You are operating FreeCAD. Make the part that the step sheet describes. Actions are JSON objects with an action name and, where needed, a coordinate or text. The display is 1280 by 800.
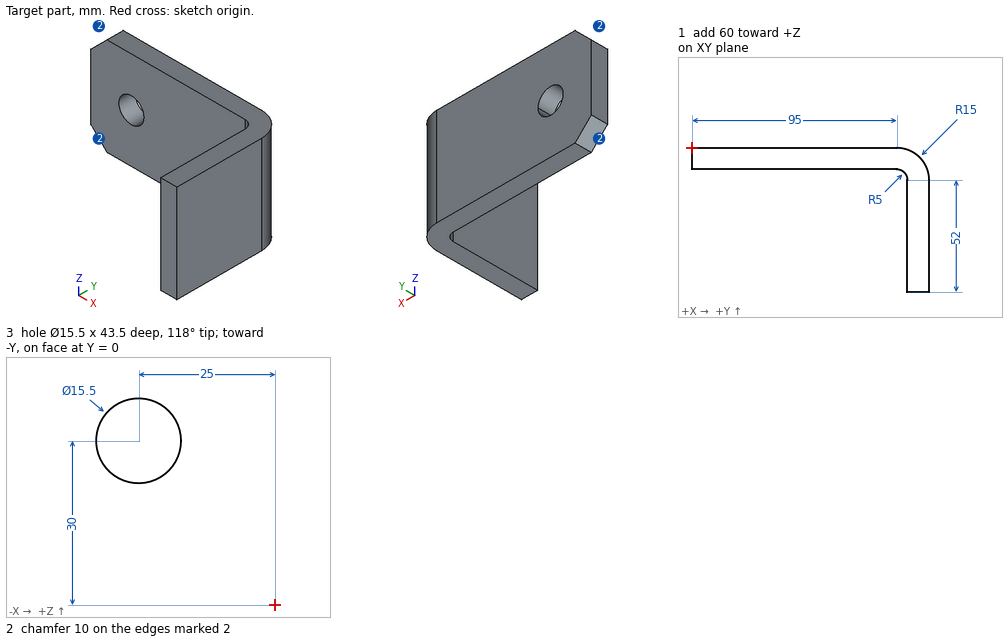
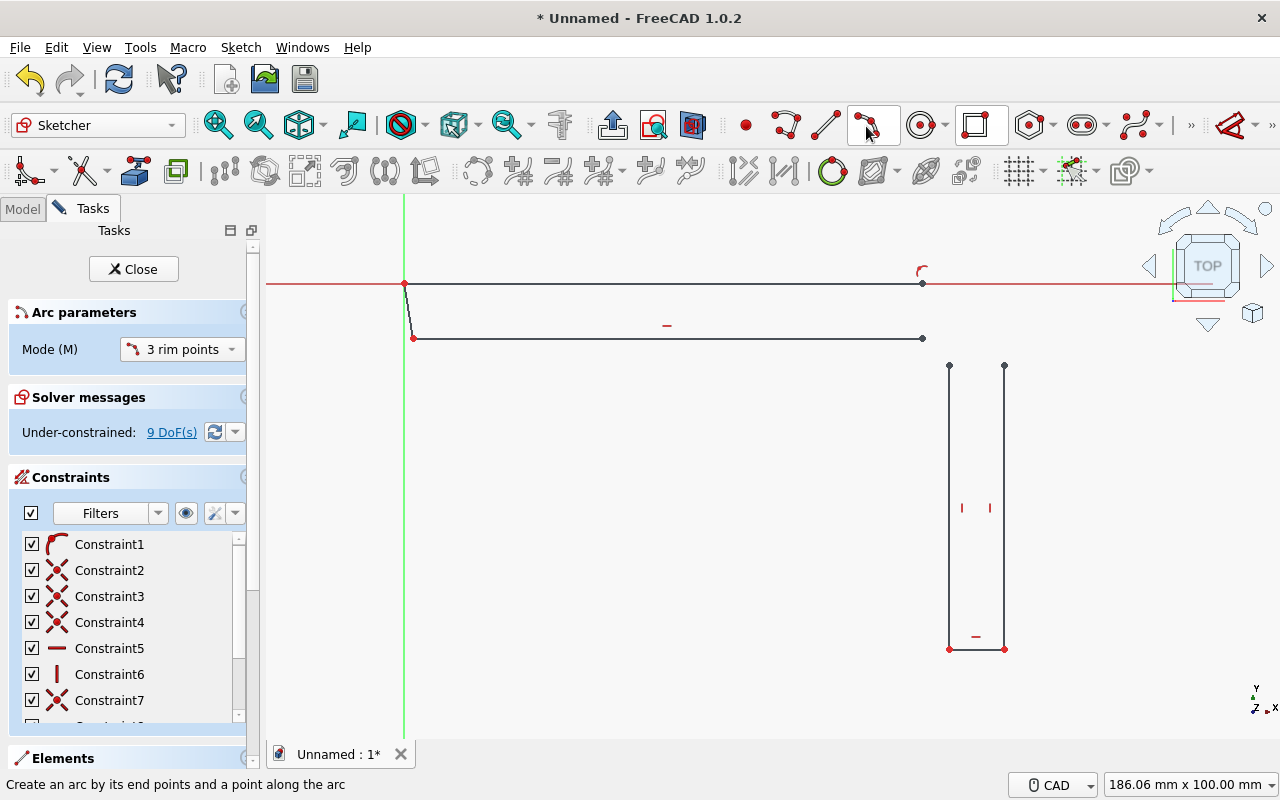
{"action": "left_click", "coordinate": [922, 339]}
{"action": "left_click", "coordinate": [949, 366]}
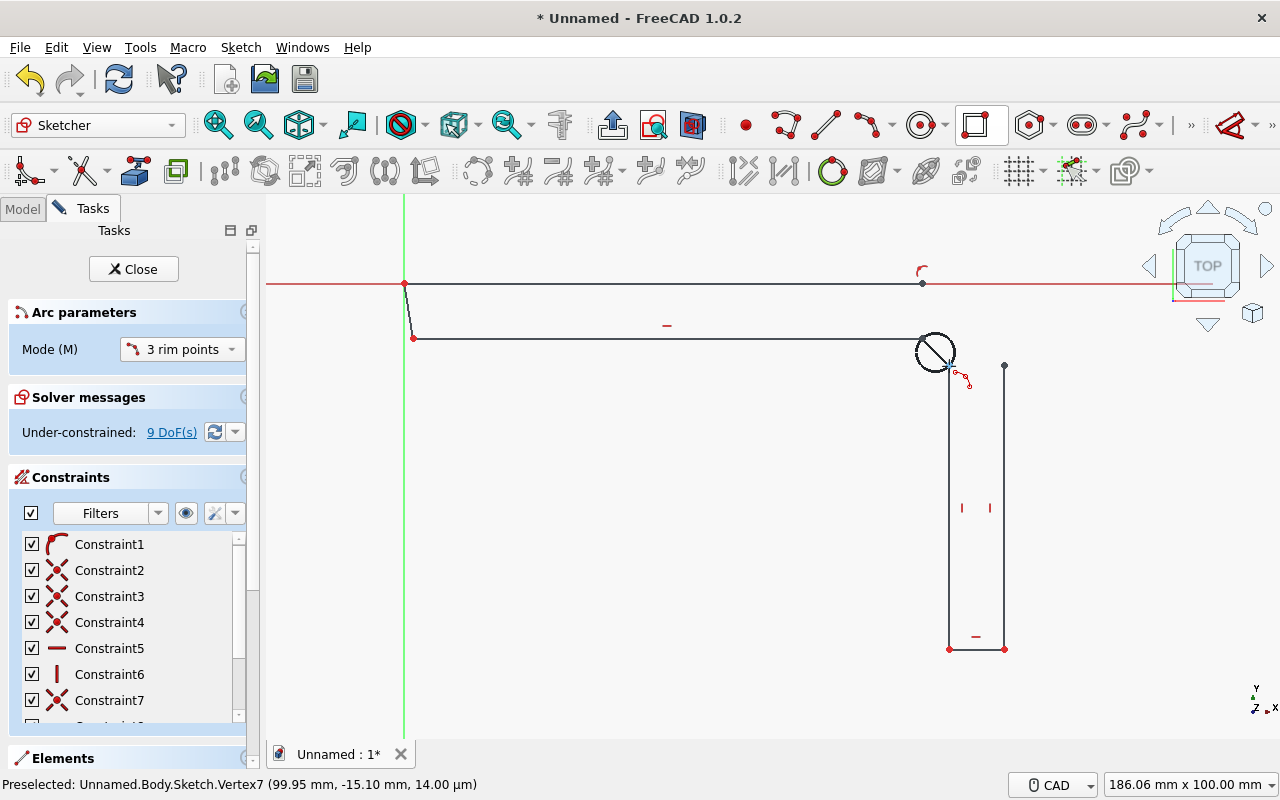
{"action": "scroll", "coordinate": [941, 346], "scroll_direction": "up", "scroll_amount": 4}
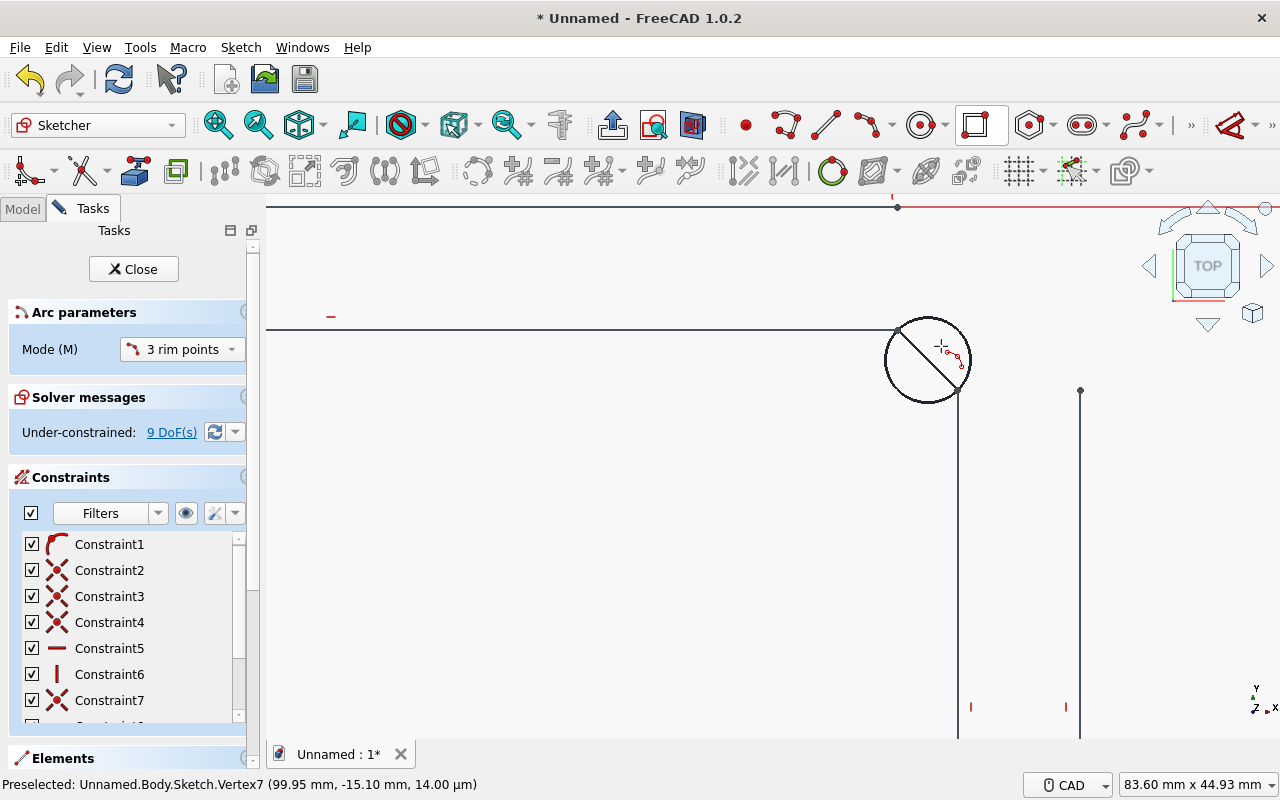
{"action": "left_click", "coordinate": [941, 346]}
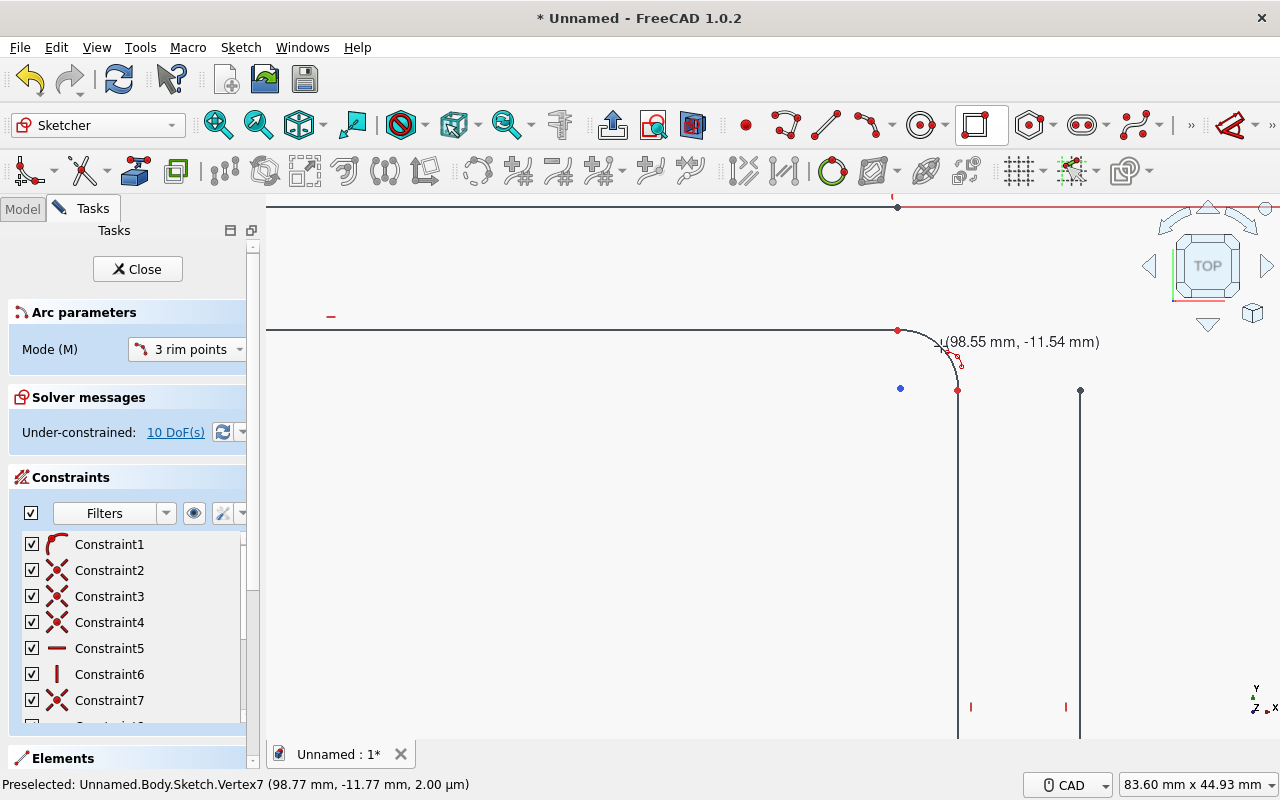
{"action": "left_click", "coordinate": [1080, 390]}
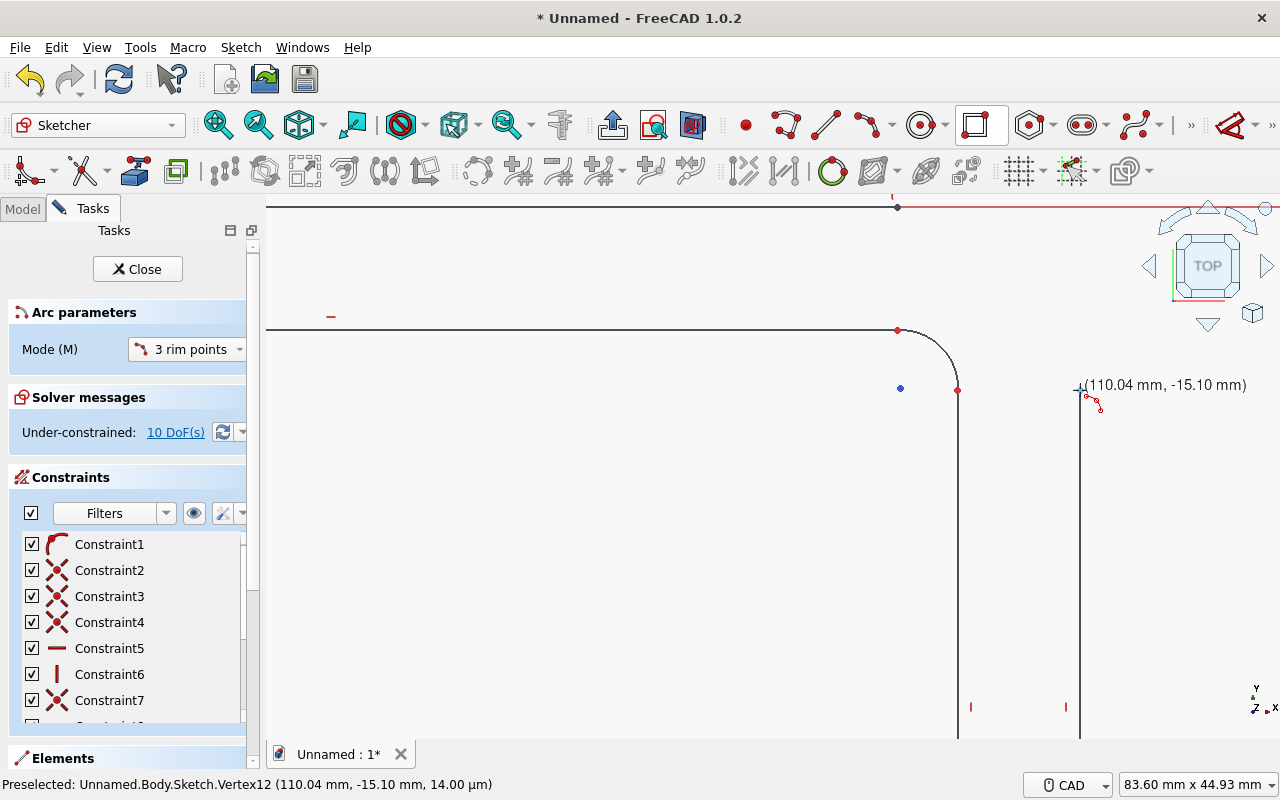
{"action": "scroll", "coordinate": [943, 347], "scroll_direction": "down", "scroll_amount": 4}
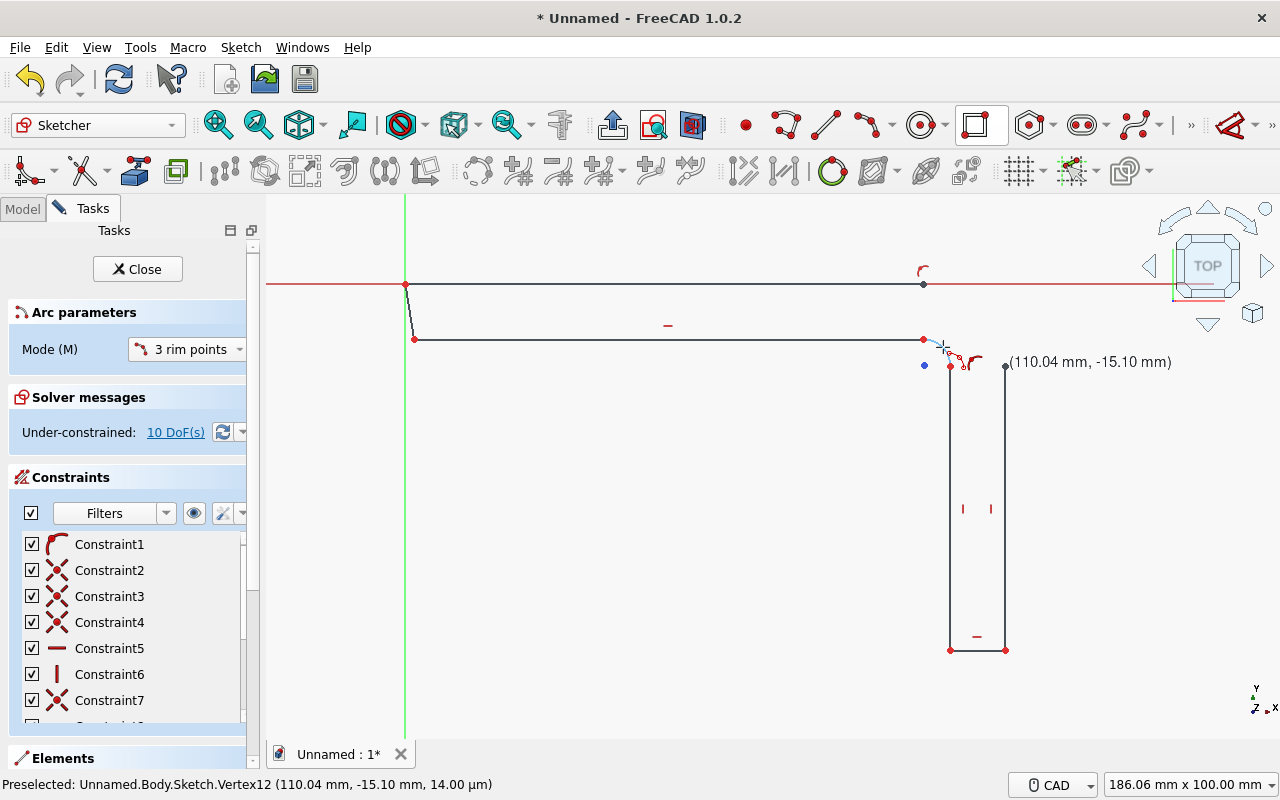
{"action": "left_click", "coordinate": [923, 284]}
{"action": "left_click", "coordinate": [981, 308]}
{"action": "key", "text": "Escape"}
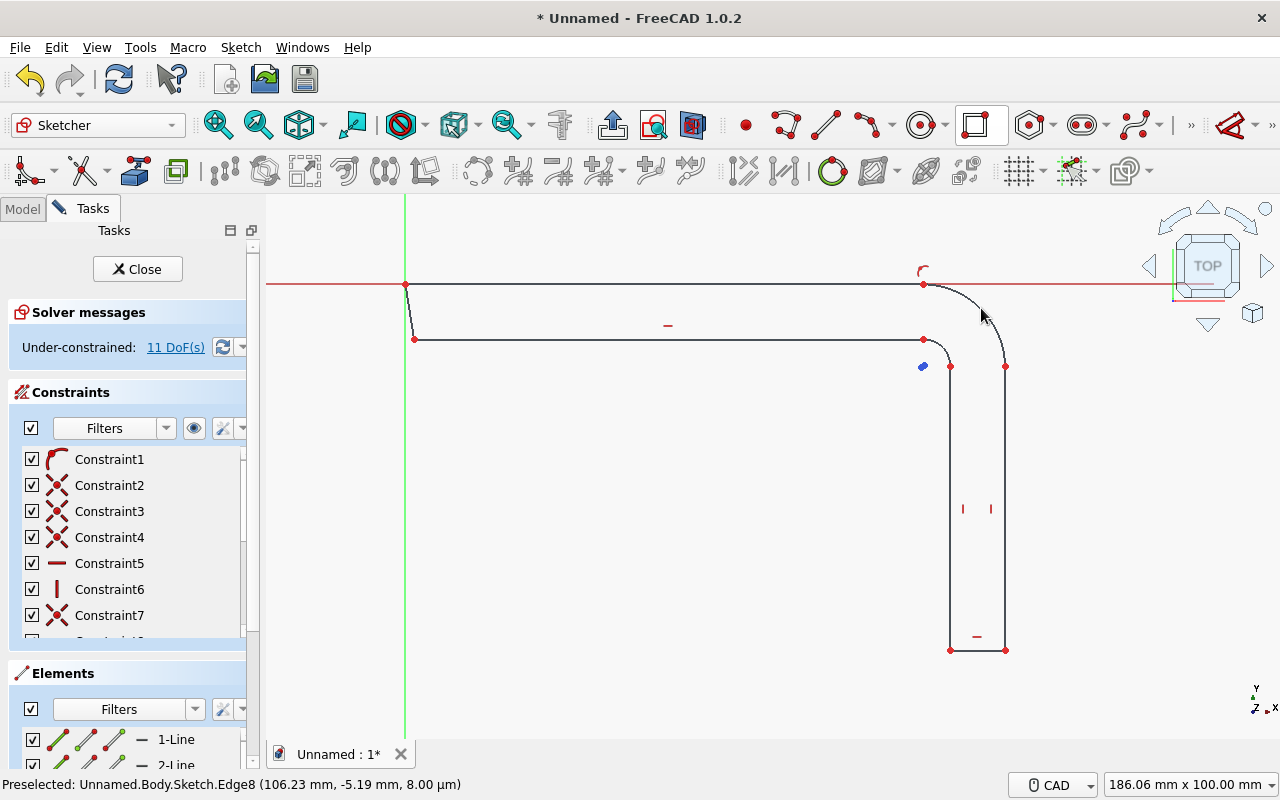
{"action": "left_click", "coordinate": [768, 284]}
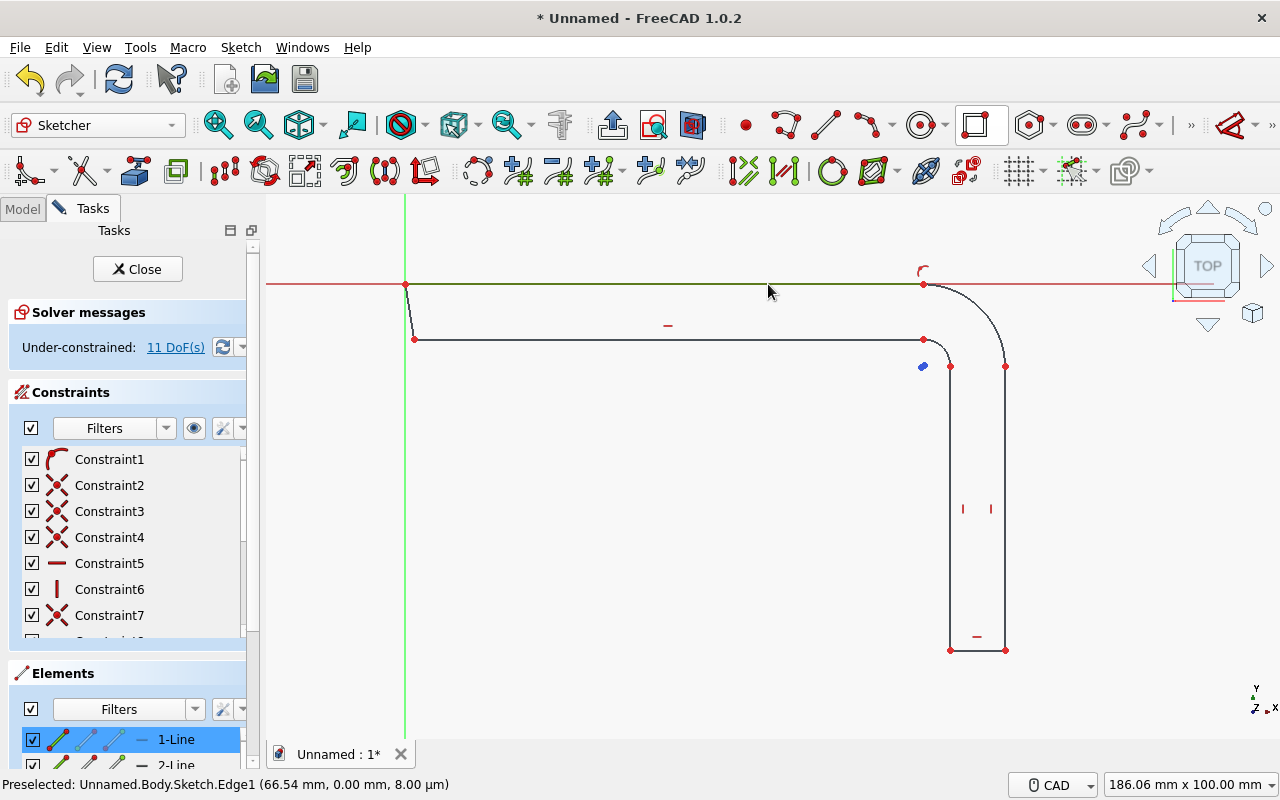
{"action": "left_click", "coordinate": [996, 329]}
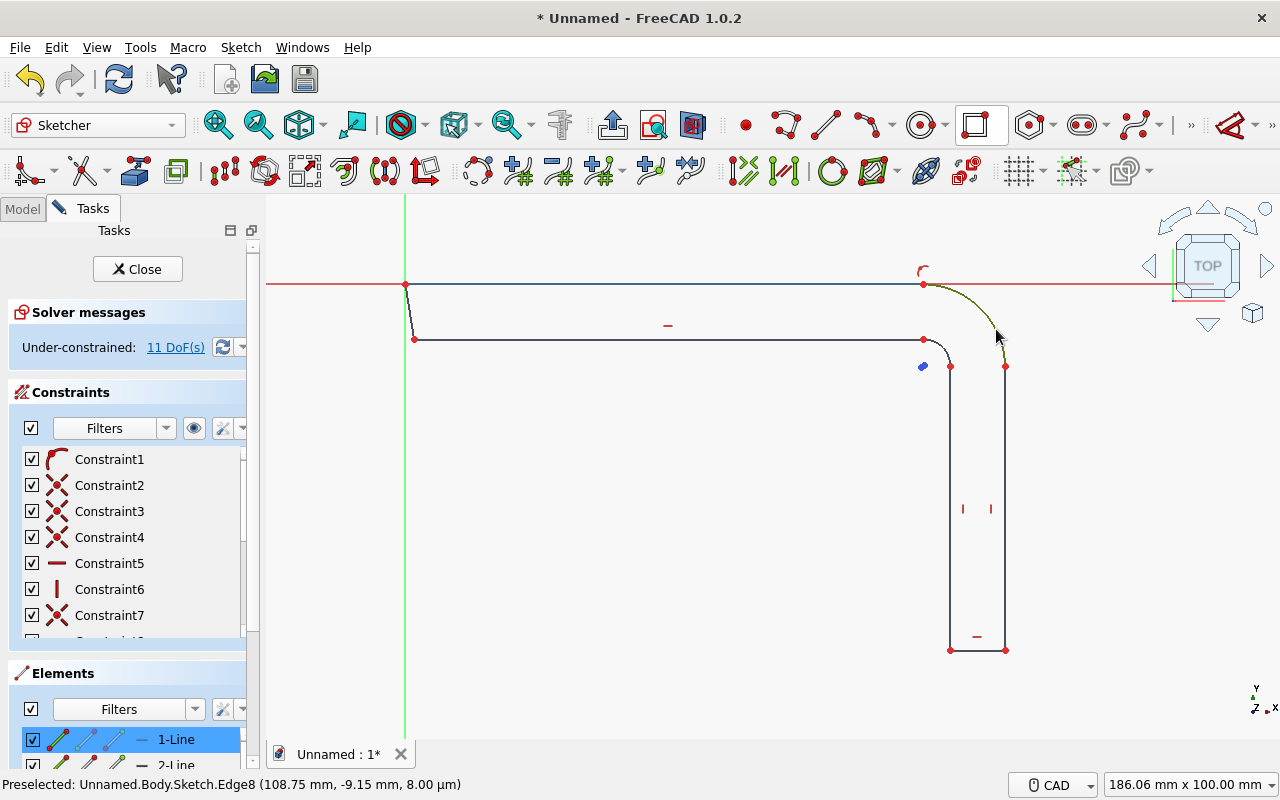
{"action": "key", "text": "t"}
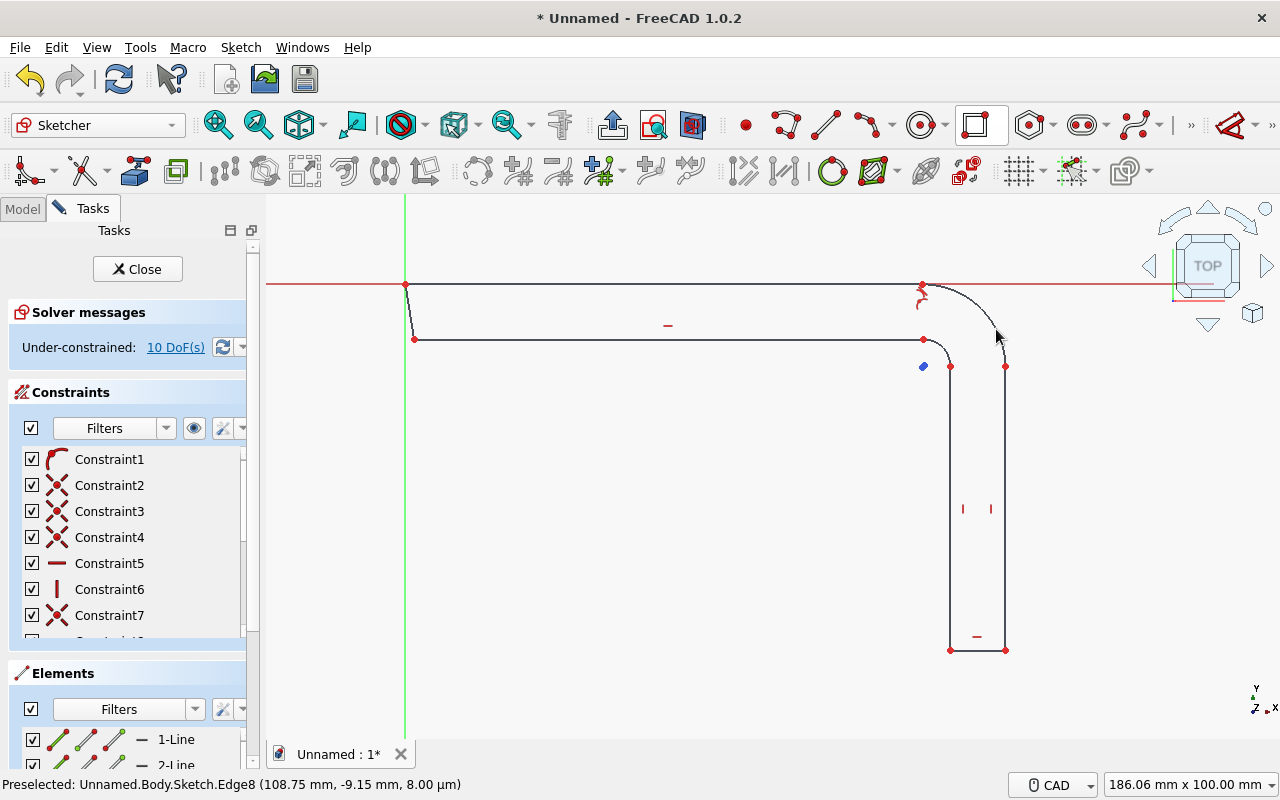
{"action": "left_click", "coordinate": [567, 340]}